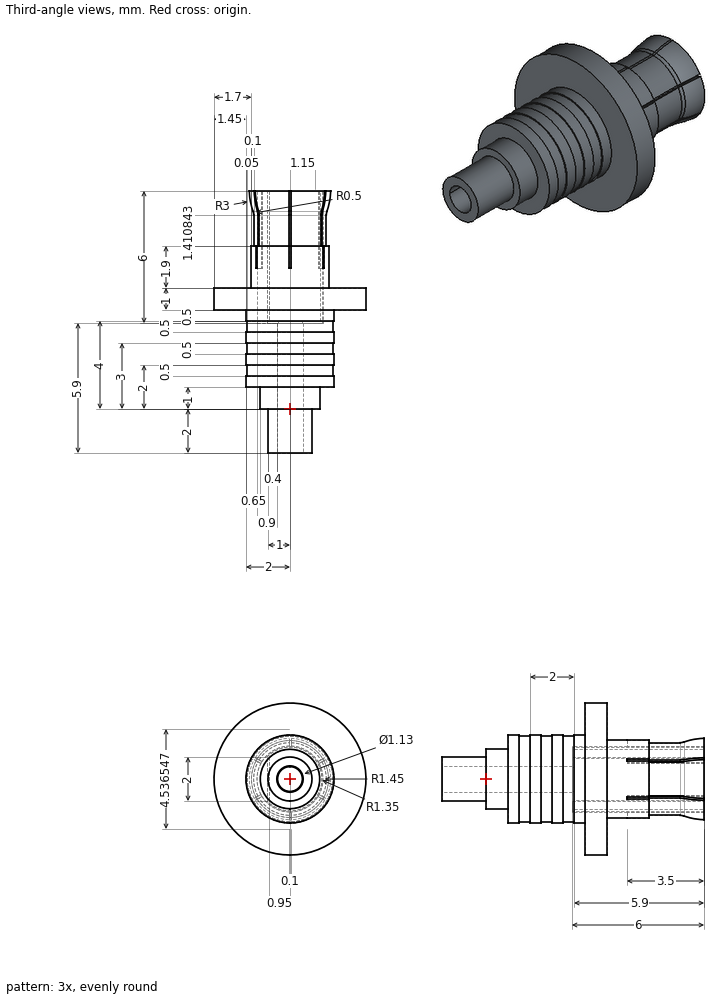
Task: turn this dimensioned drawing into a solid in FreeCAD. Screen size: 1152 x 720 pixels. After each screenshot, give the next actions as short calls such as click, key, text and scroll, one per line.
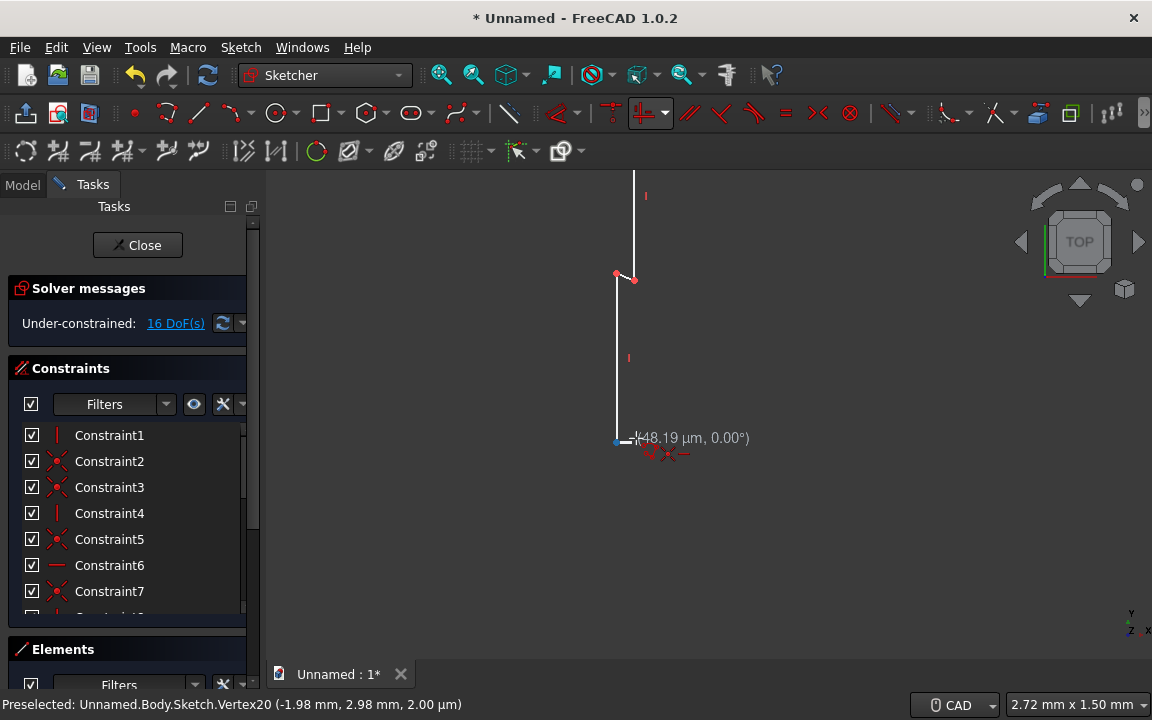
click(634, 434)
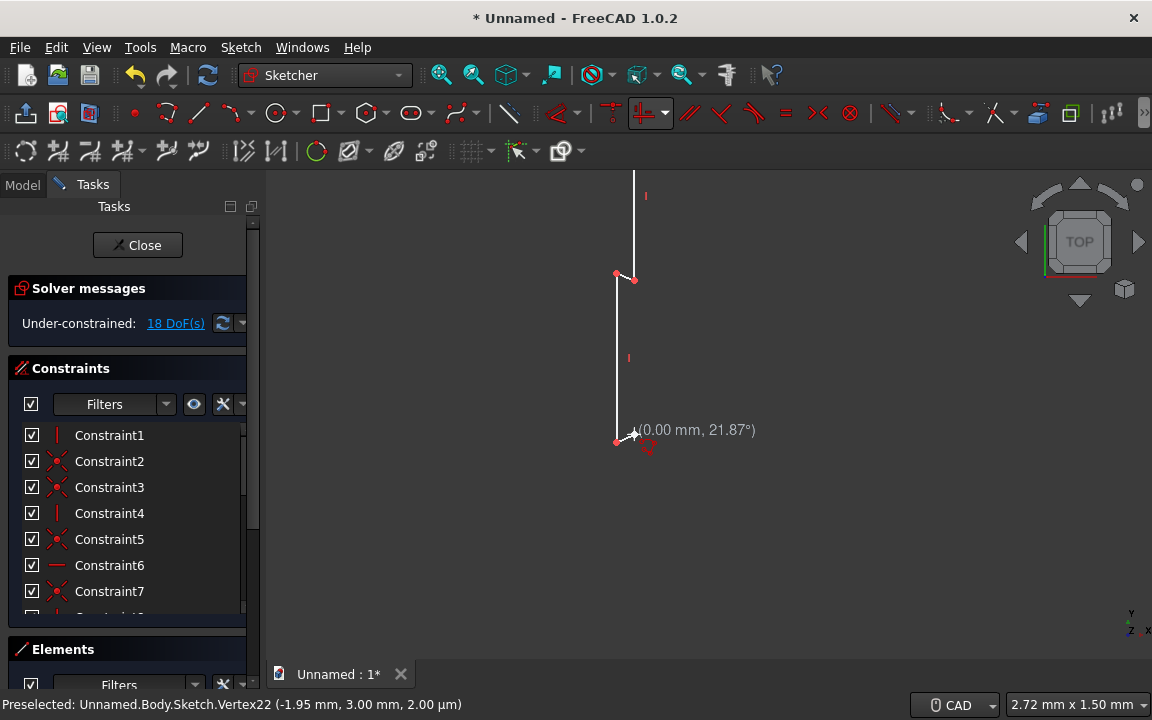
scroll(635, 438, down, 13)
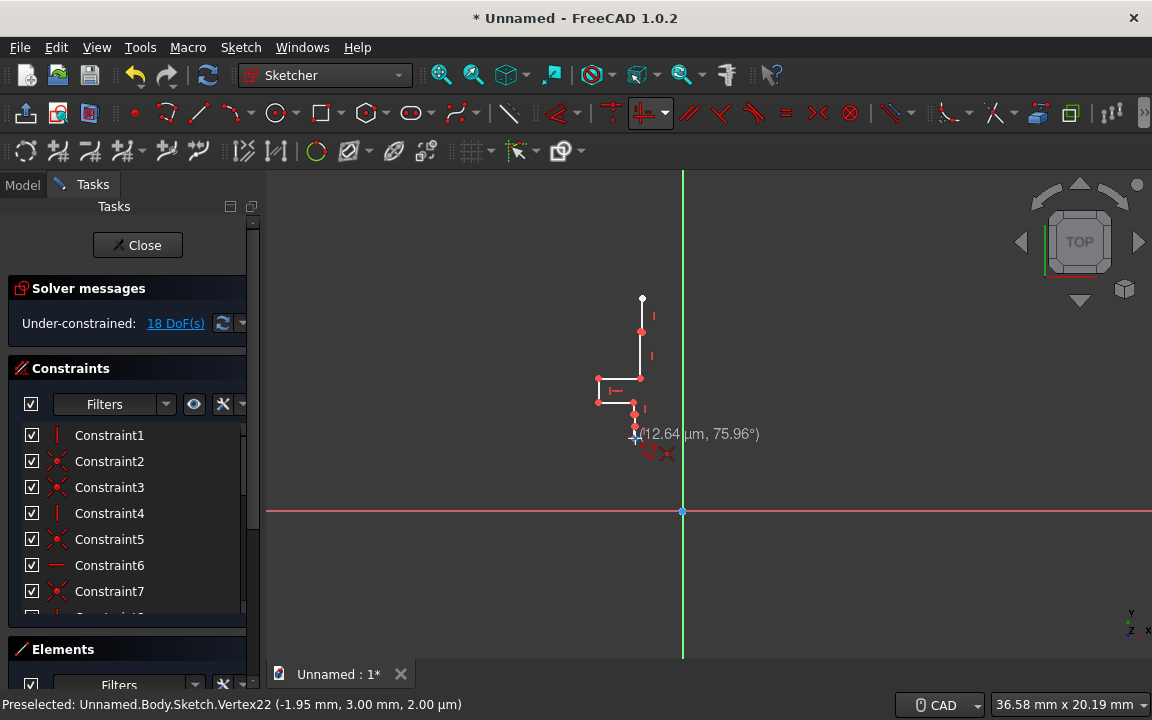
scroll(635, 450, up, 2)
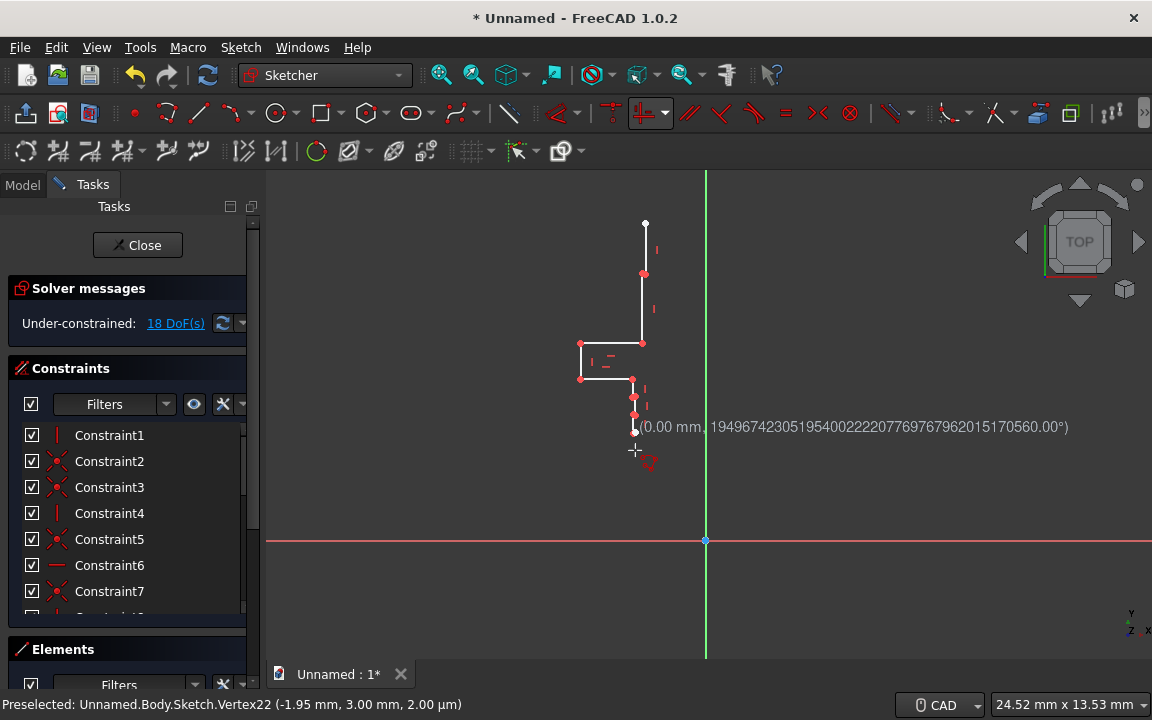
click(635, 450)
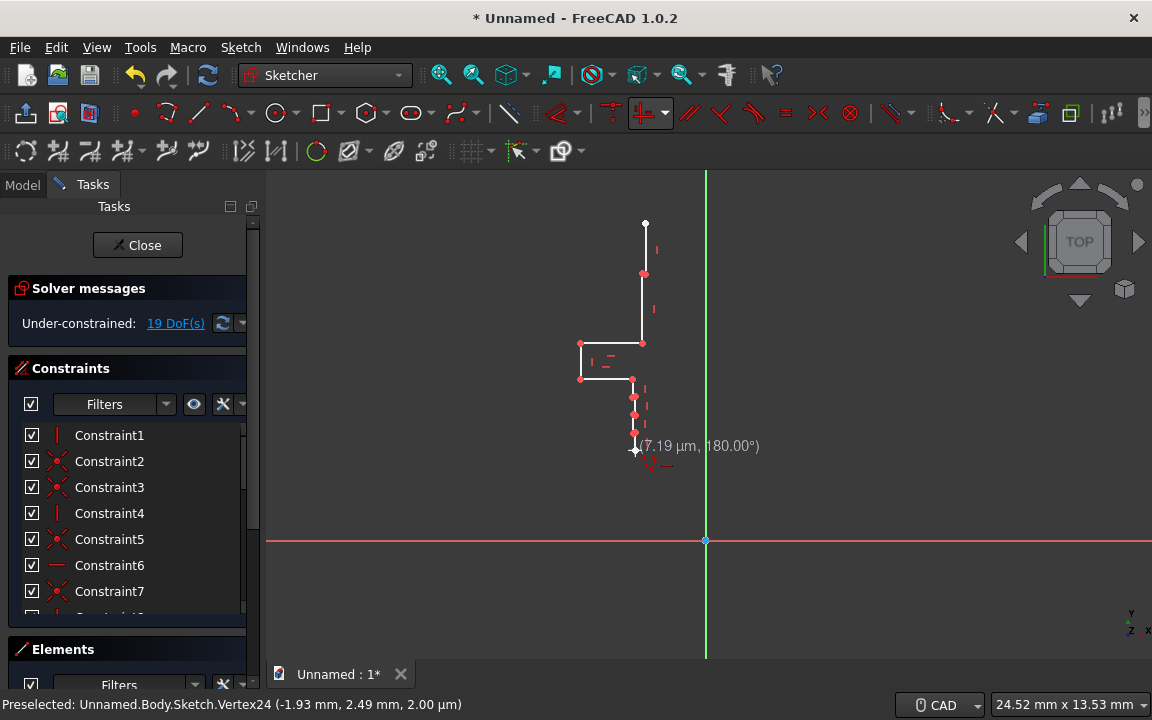
scroll(633, 450, up, 11)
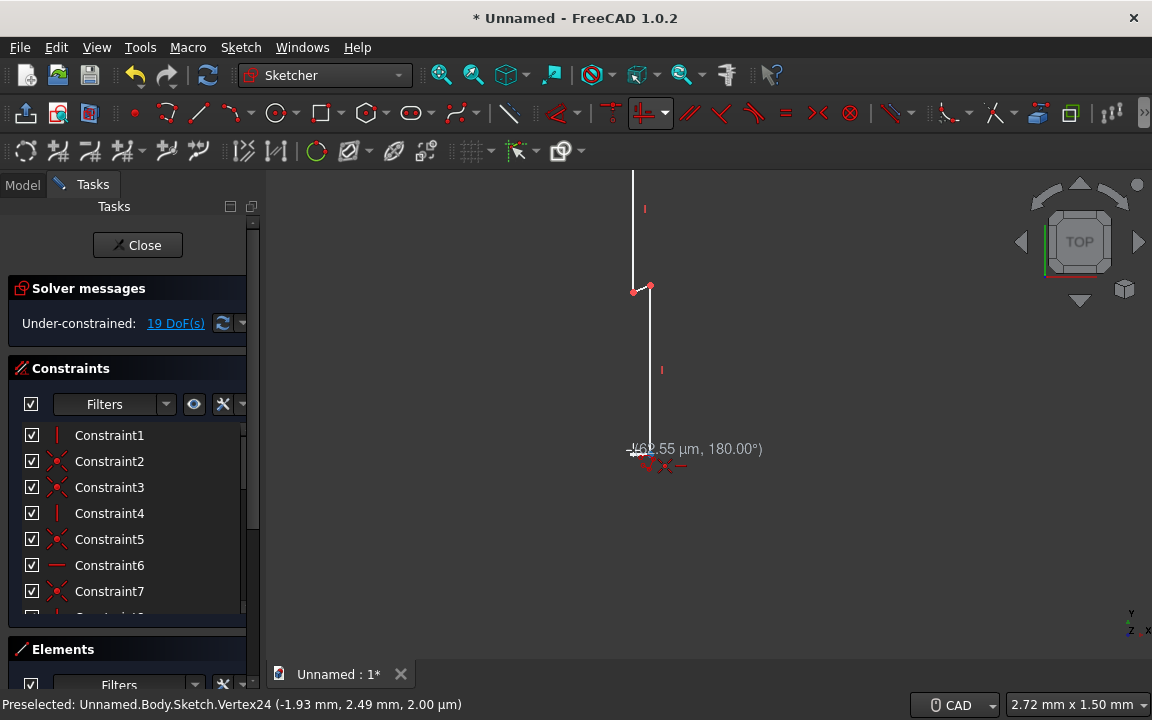
click(633, 445)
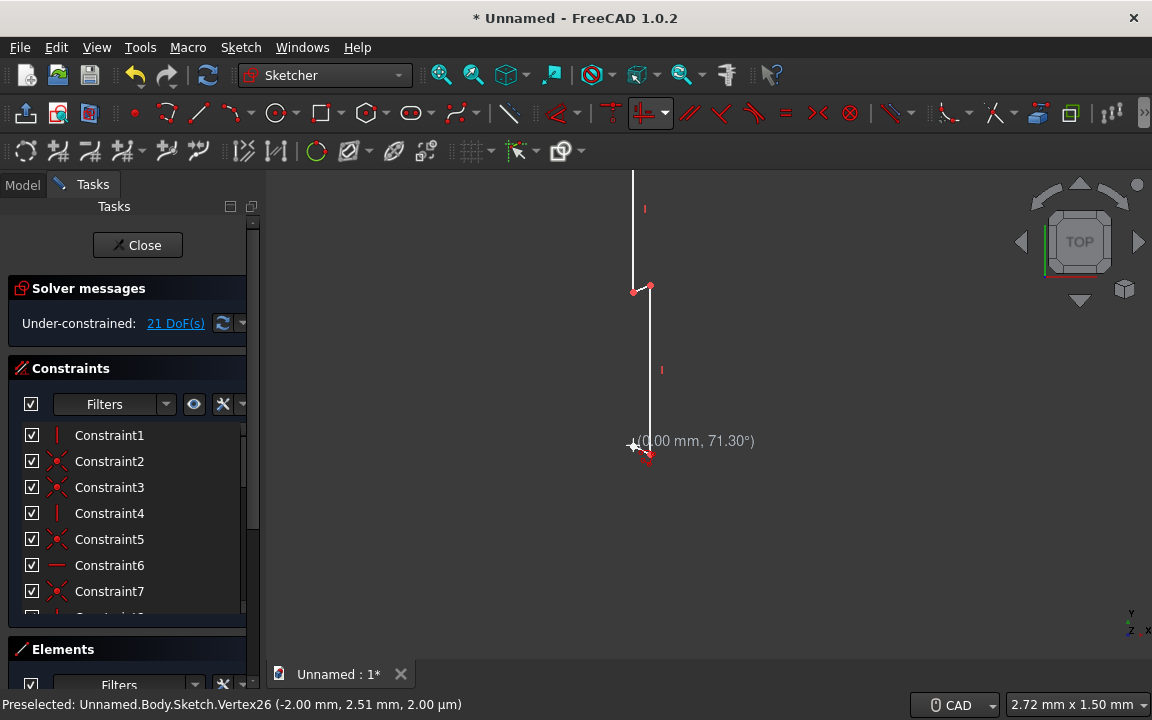
scroll(634, 450, down, 13)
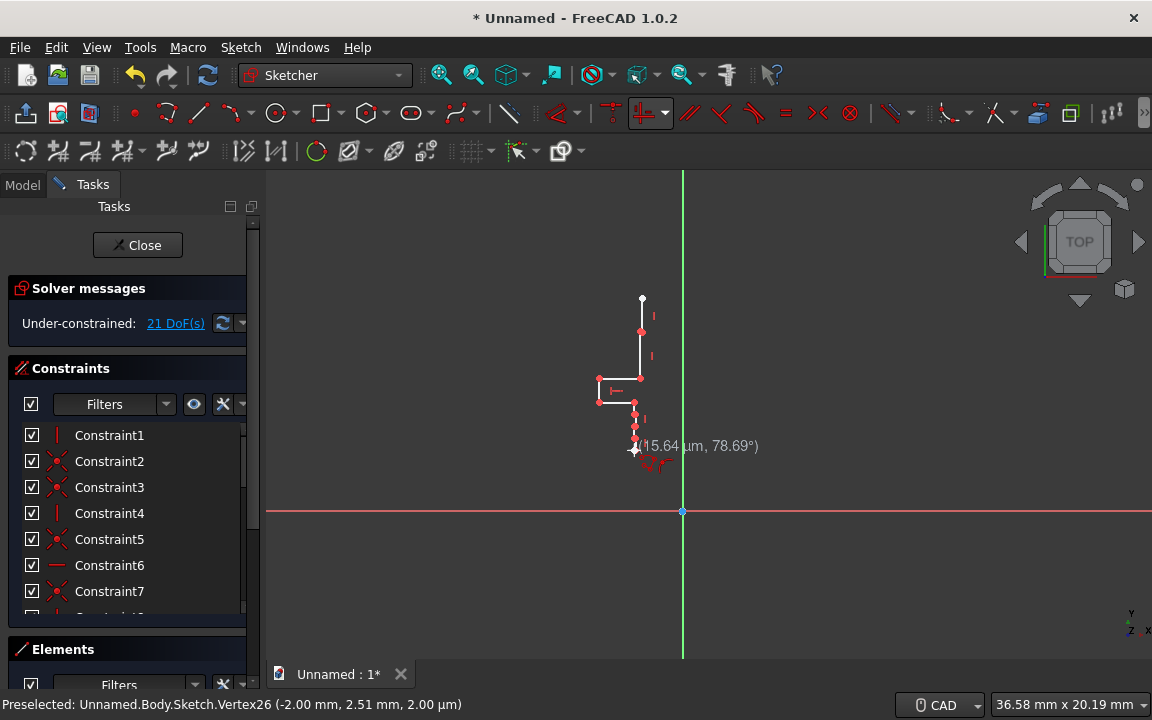
scroll(634, 463, up, 2)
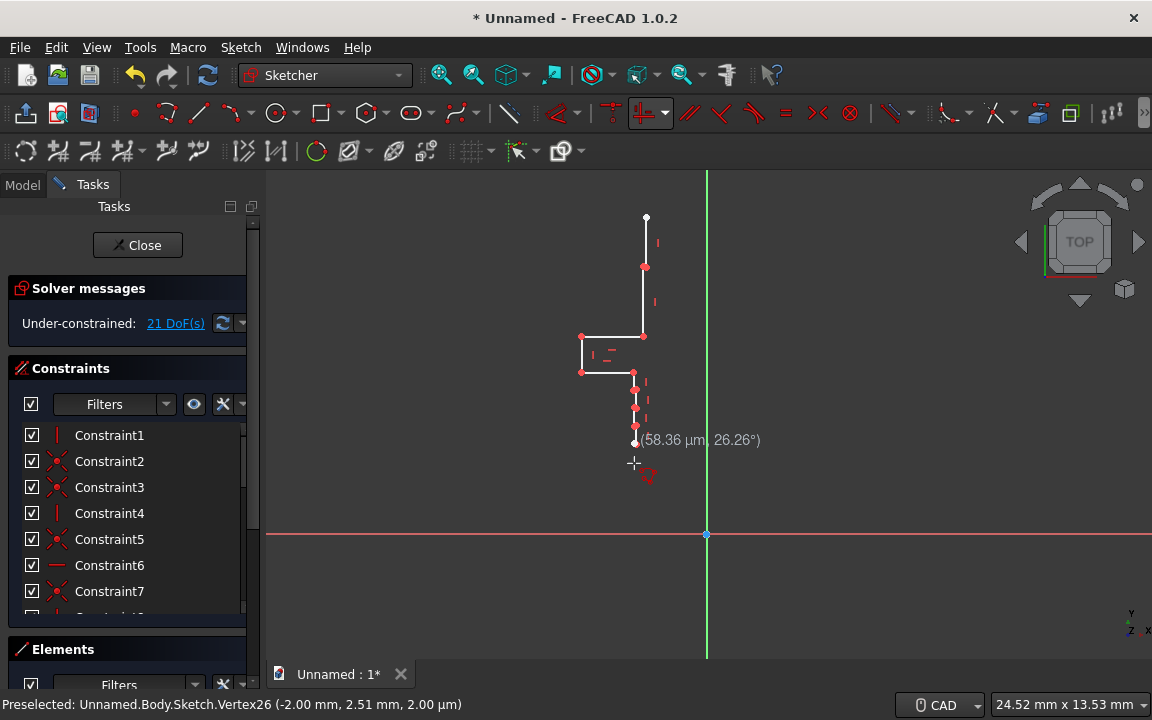
click(634, 462)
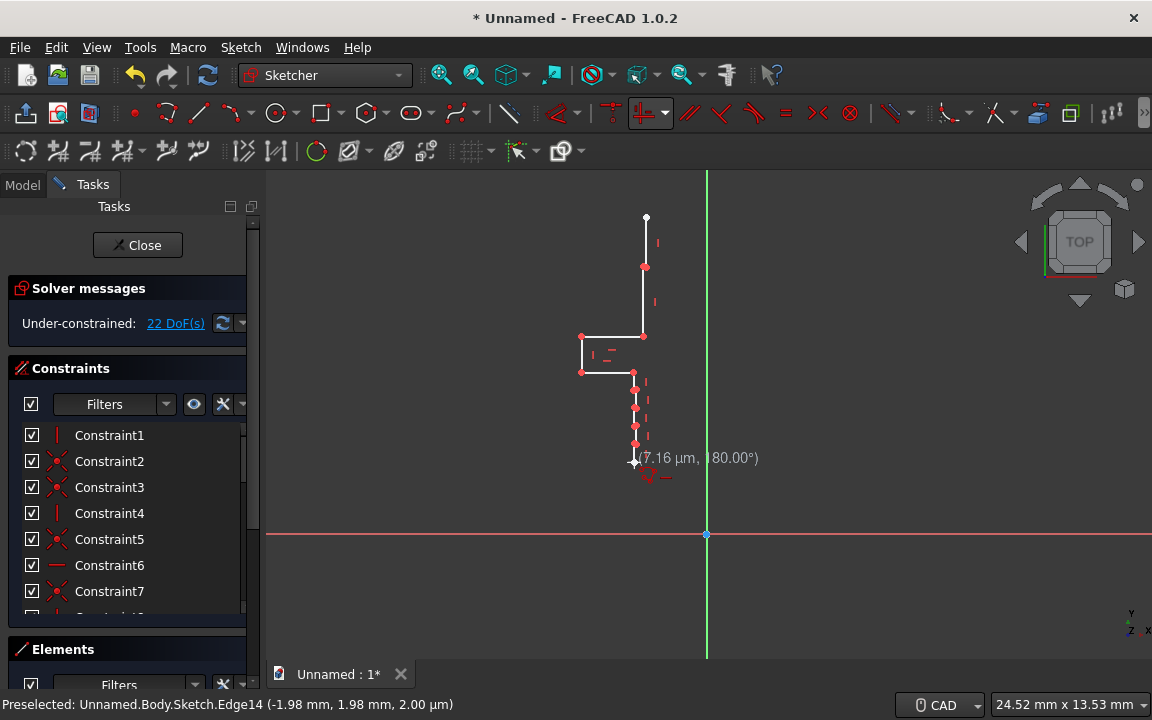
scroll(636, 462, up, 11)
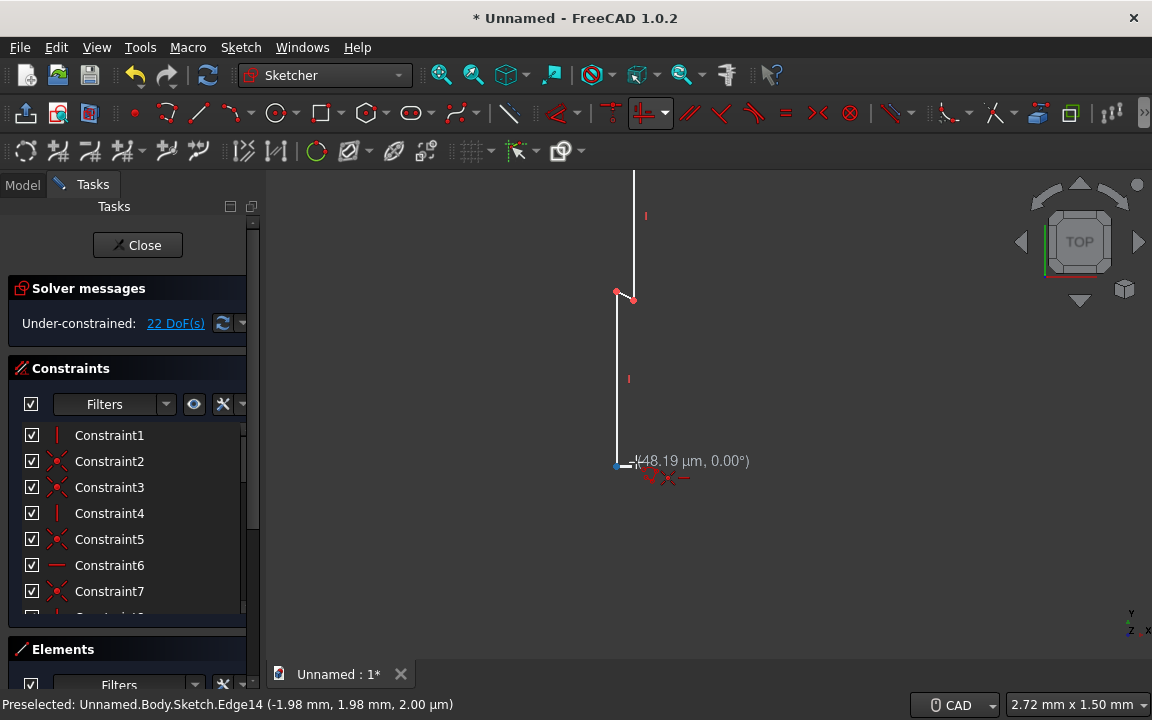
click(634, 457)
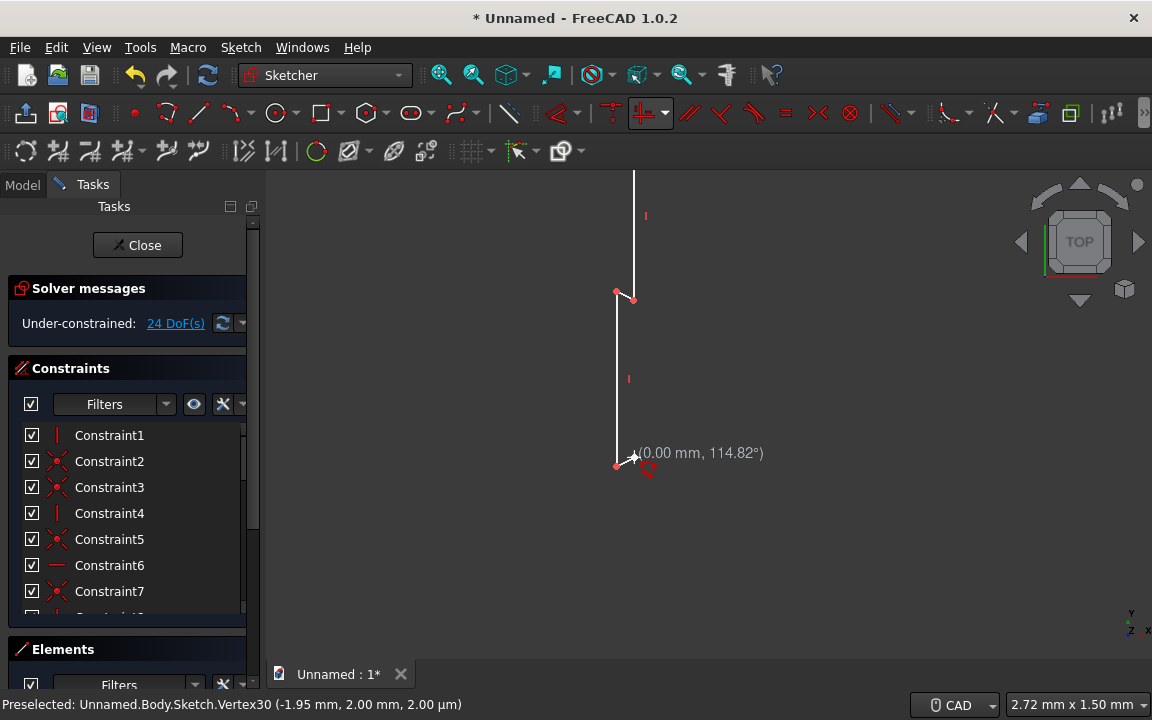
scroll(635, 462, down, 13)